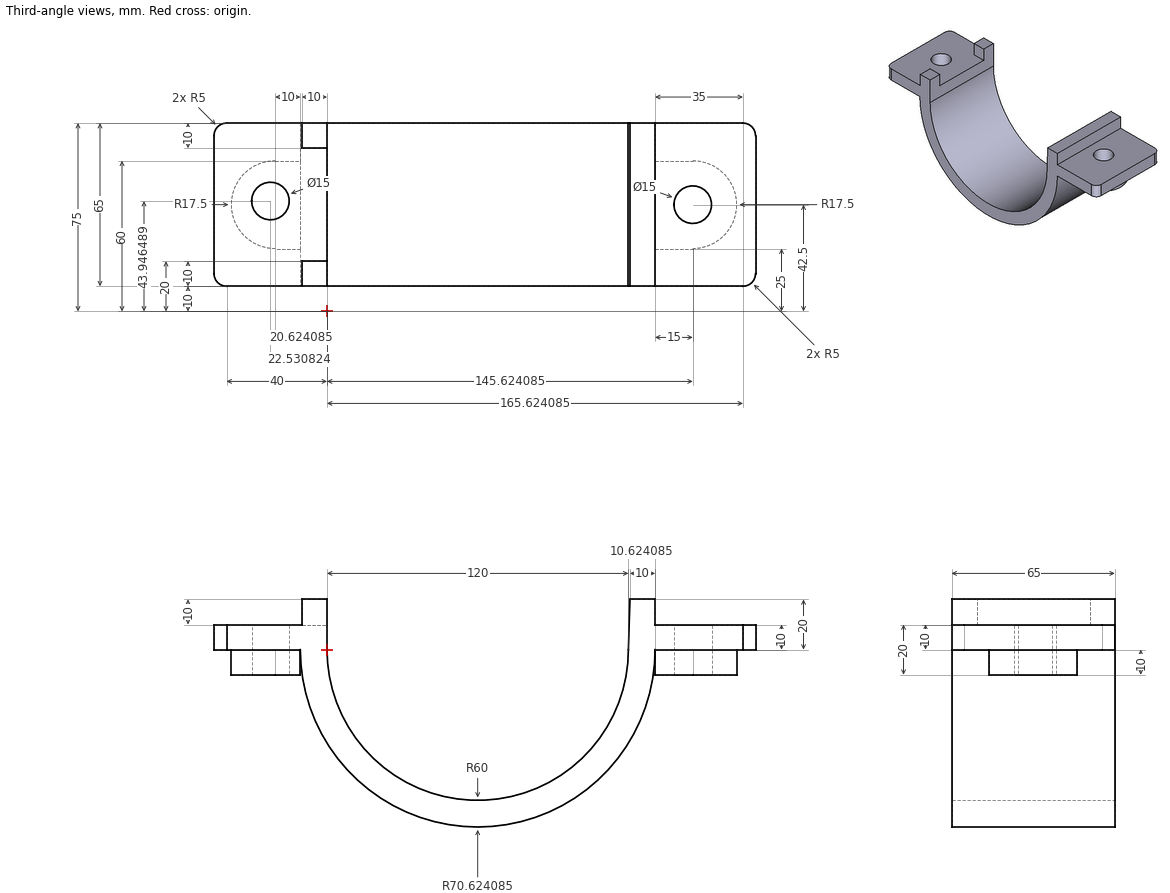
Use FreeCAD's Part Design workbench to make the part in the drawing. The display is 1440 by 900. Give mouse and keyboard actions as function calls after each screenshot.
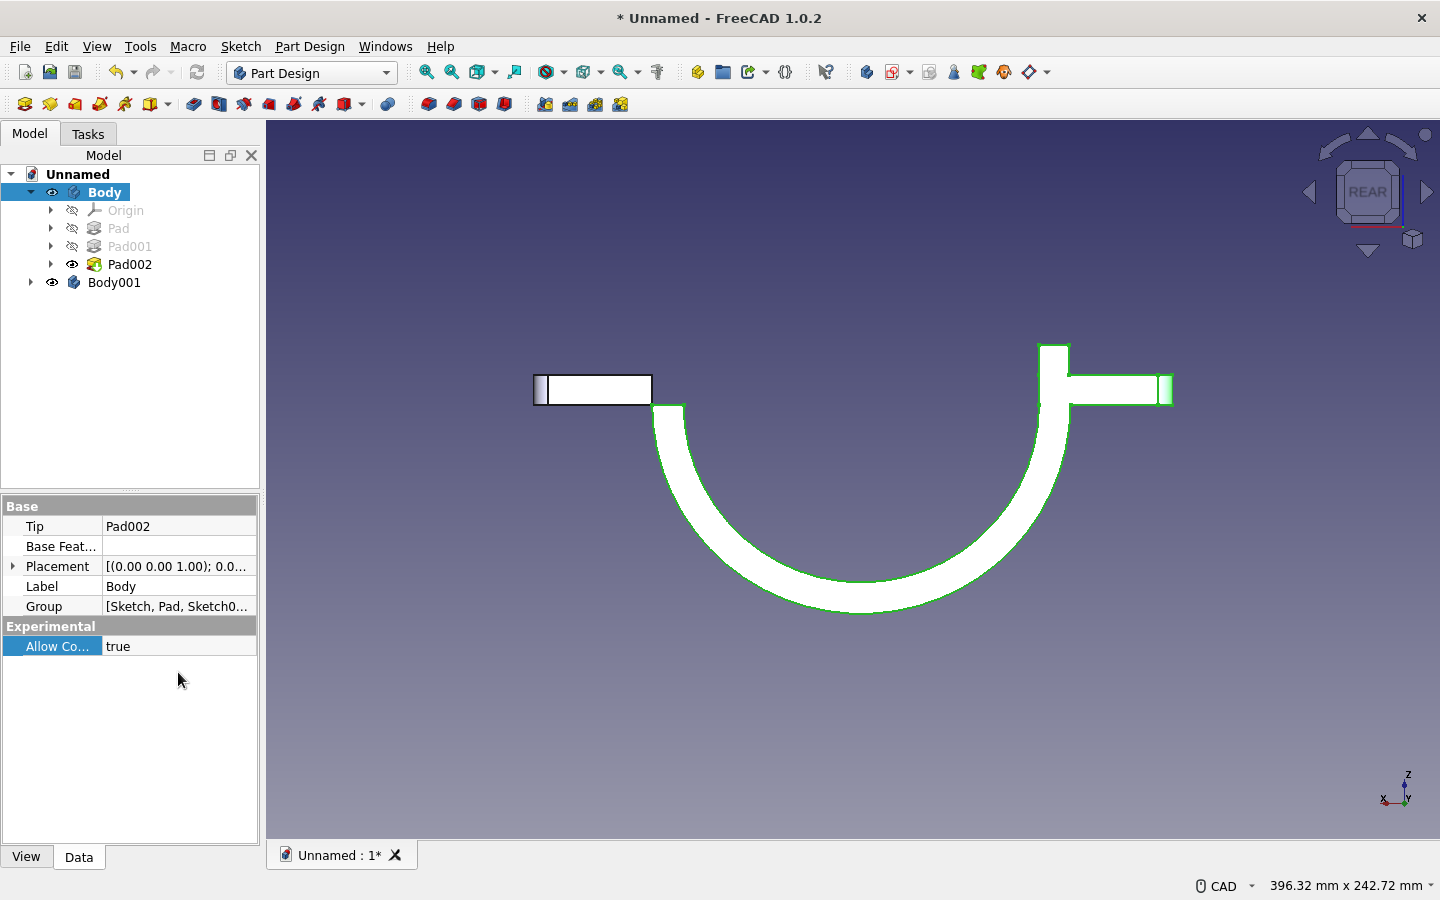
click(97, 282)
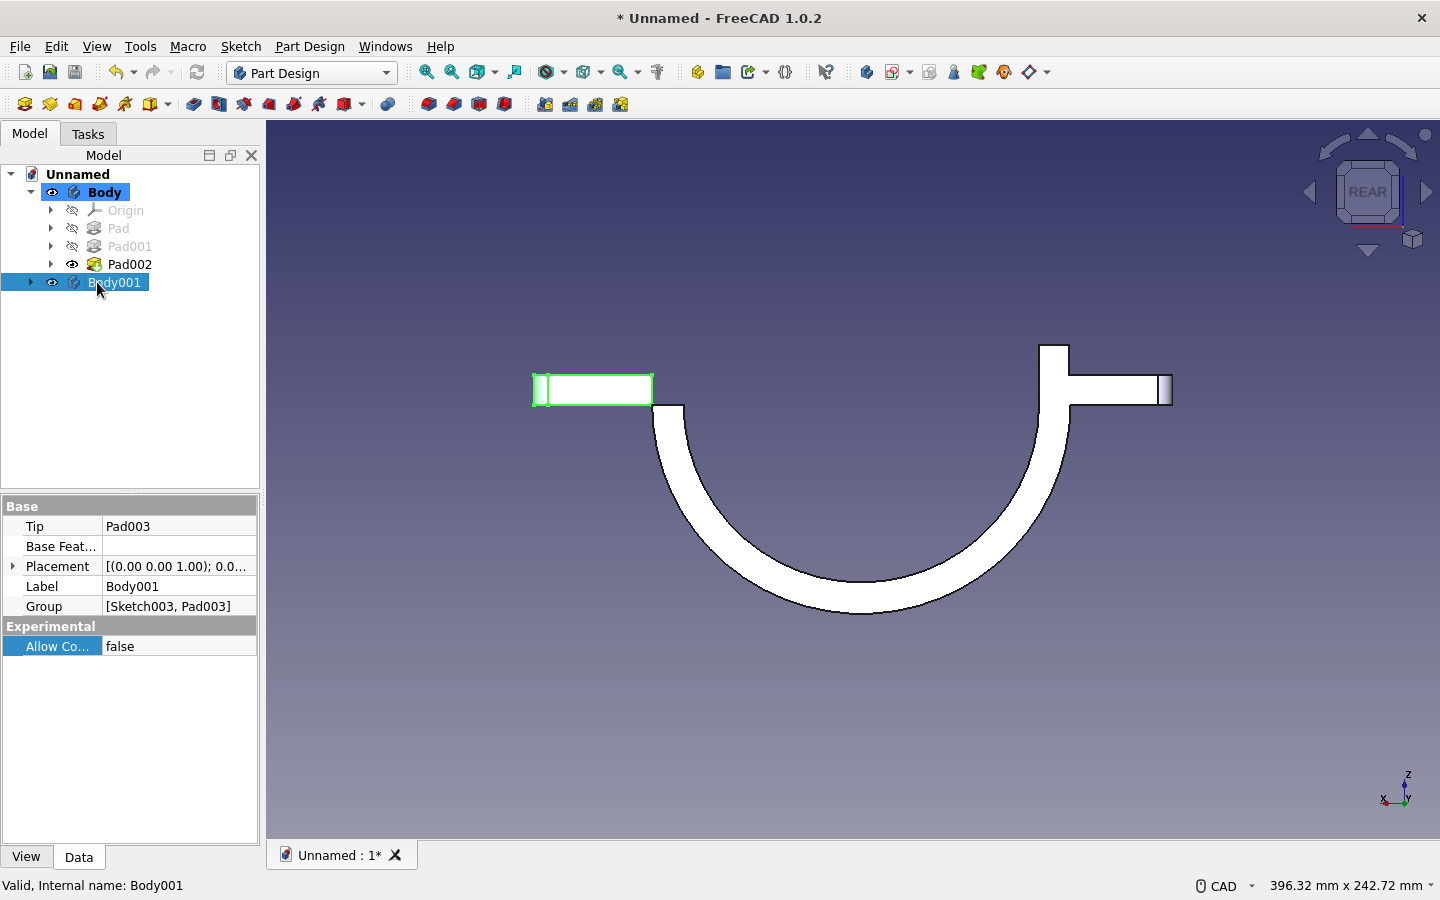
click(388, 104)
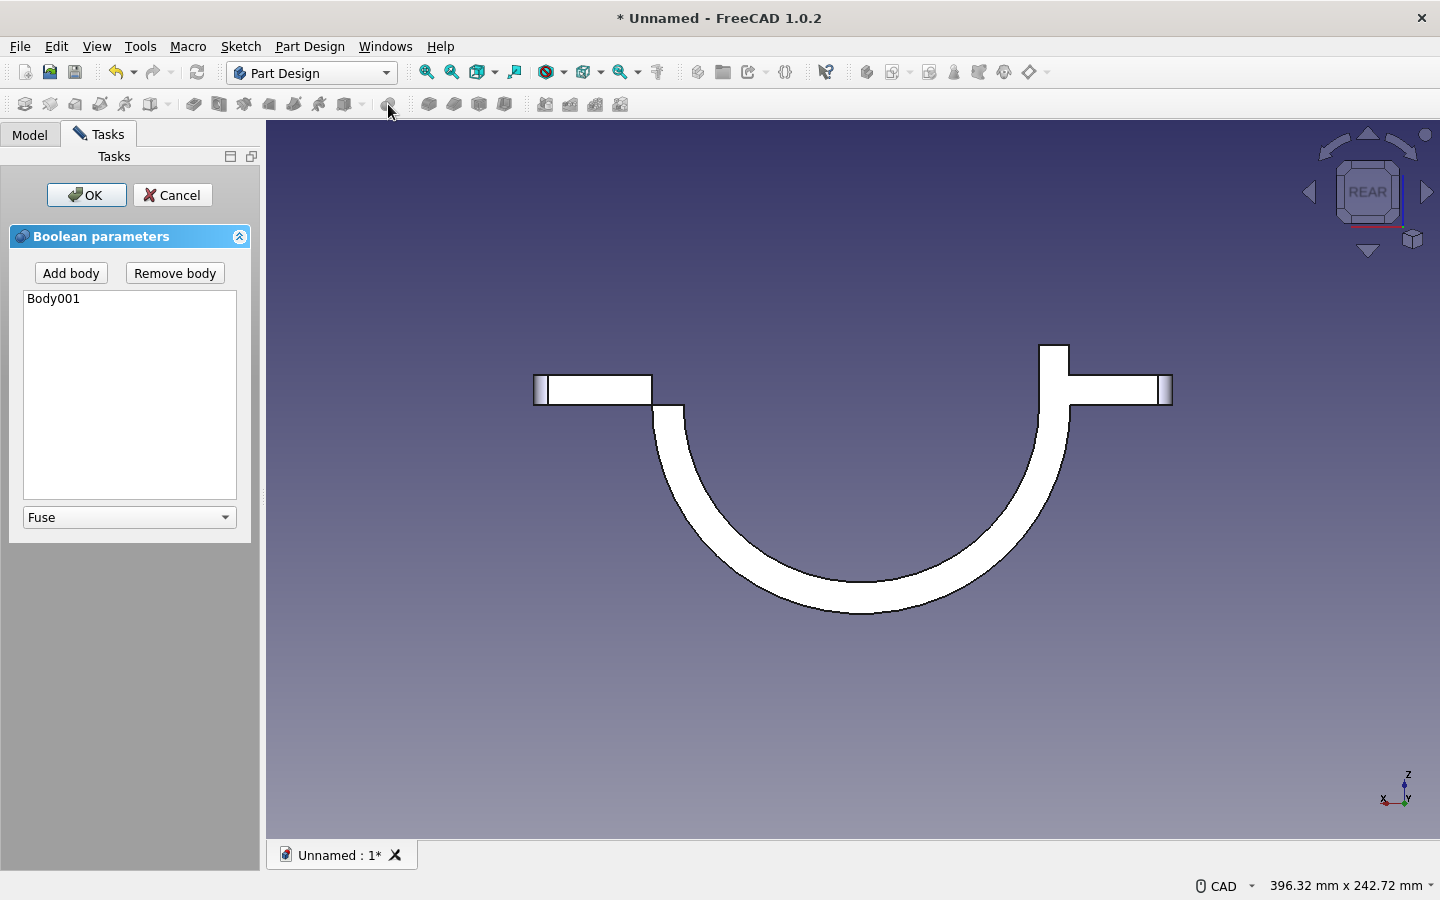
click(87, 195)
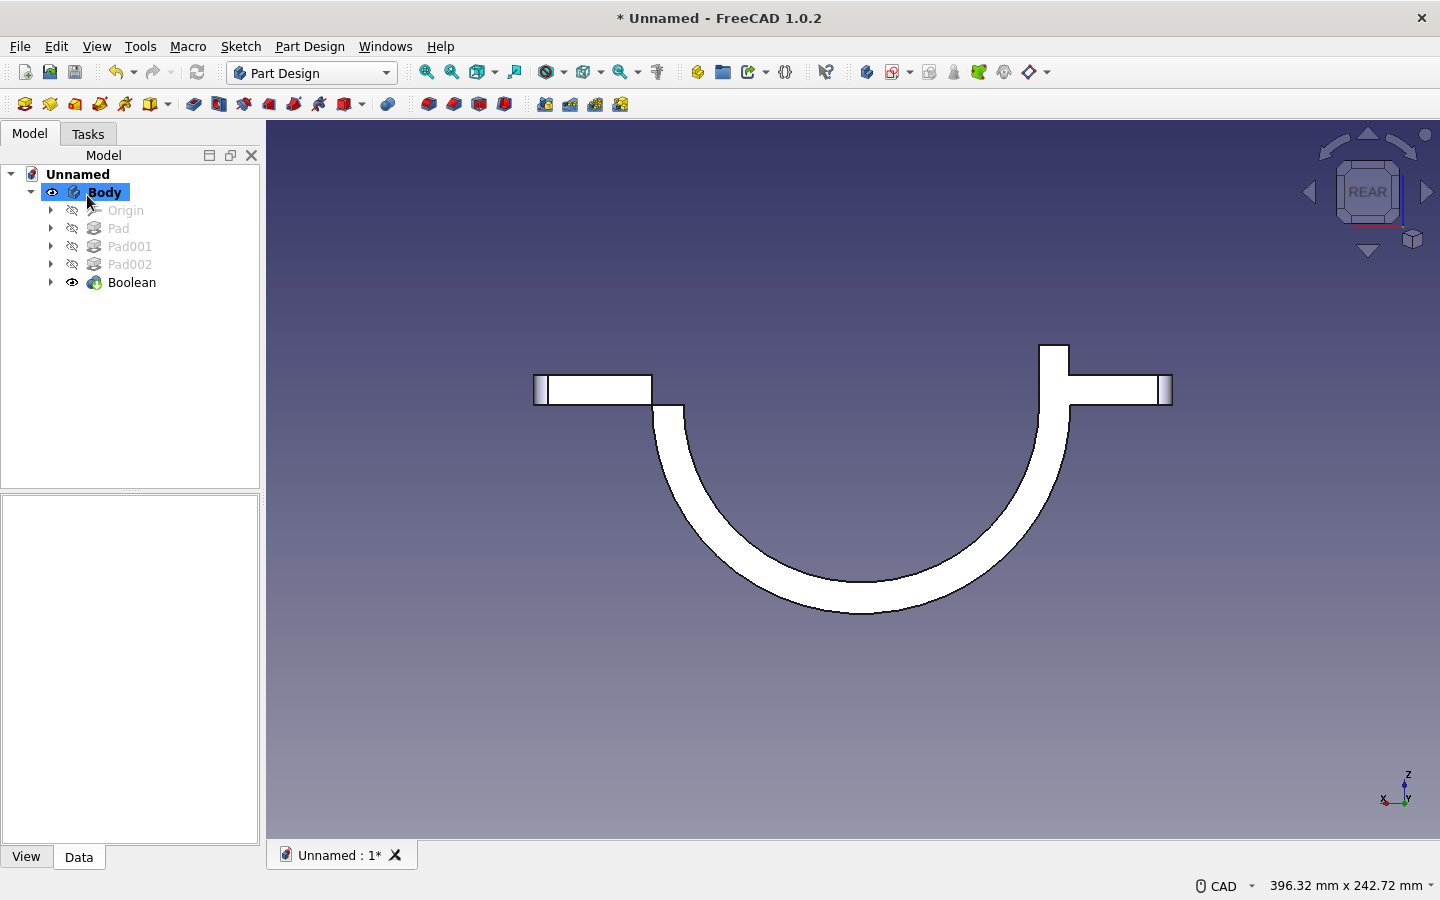
click(833, 594)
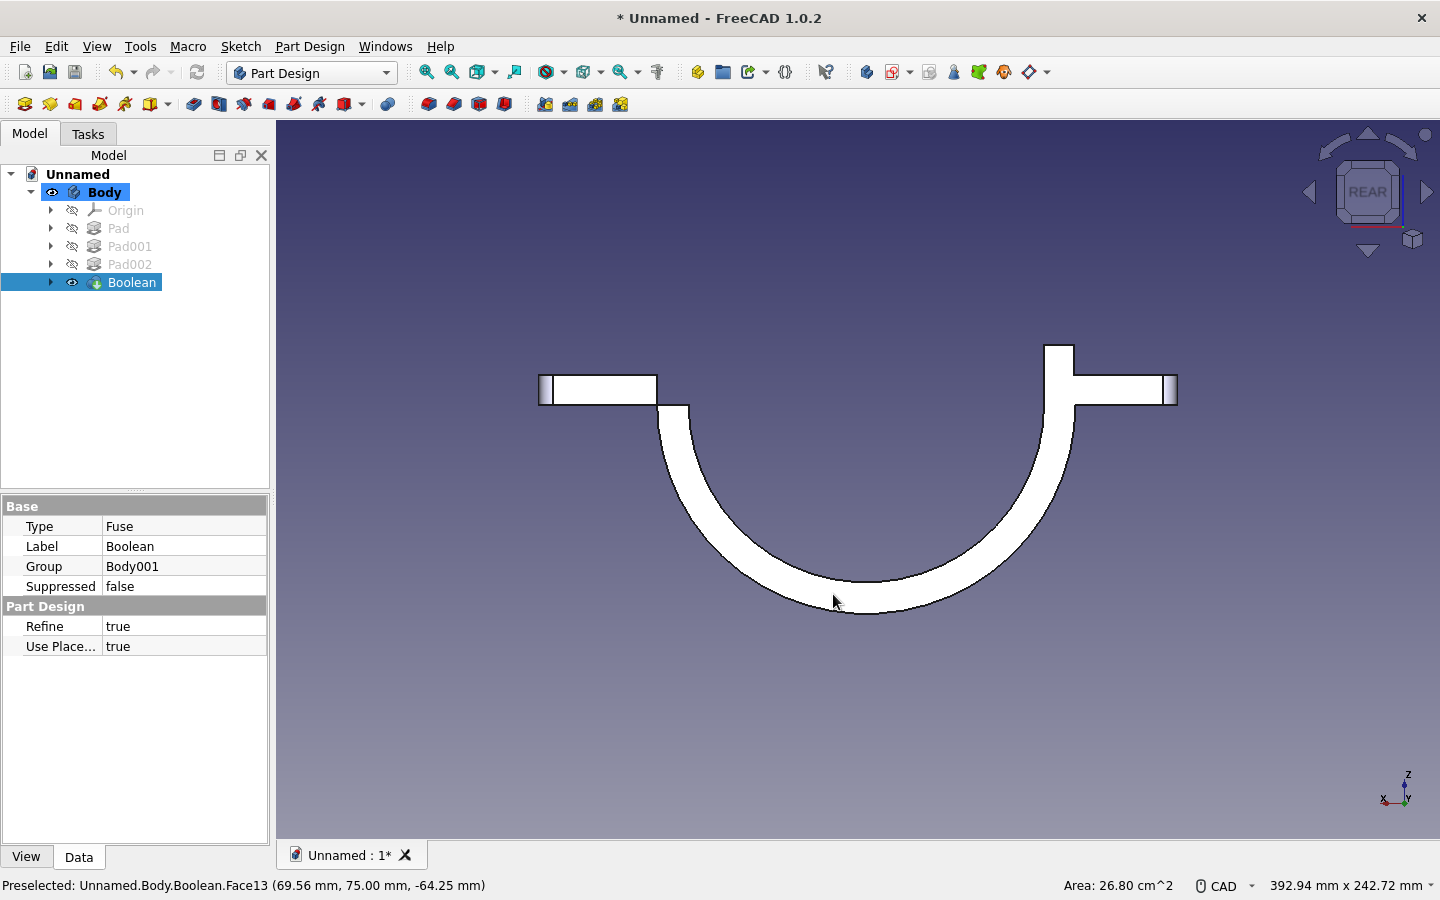
click(892, 72)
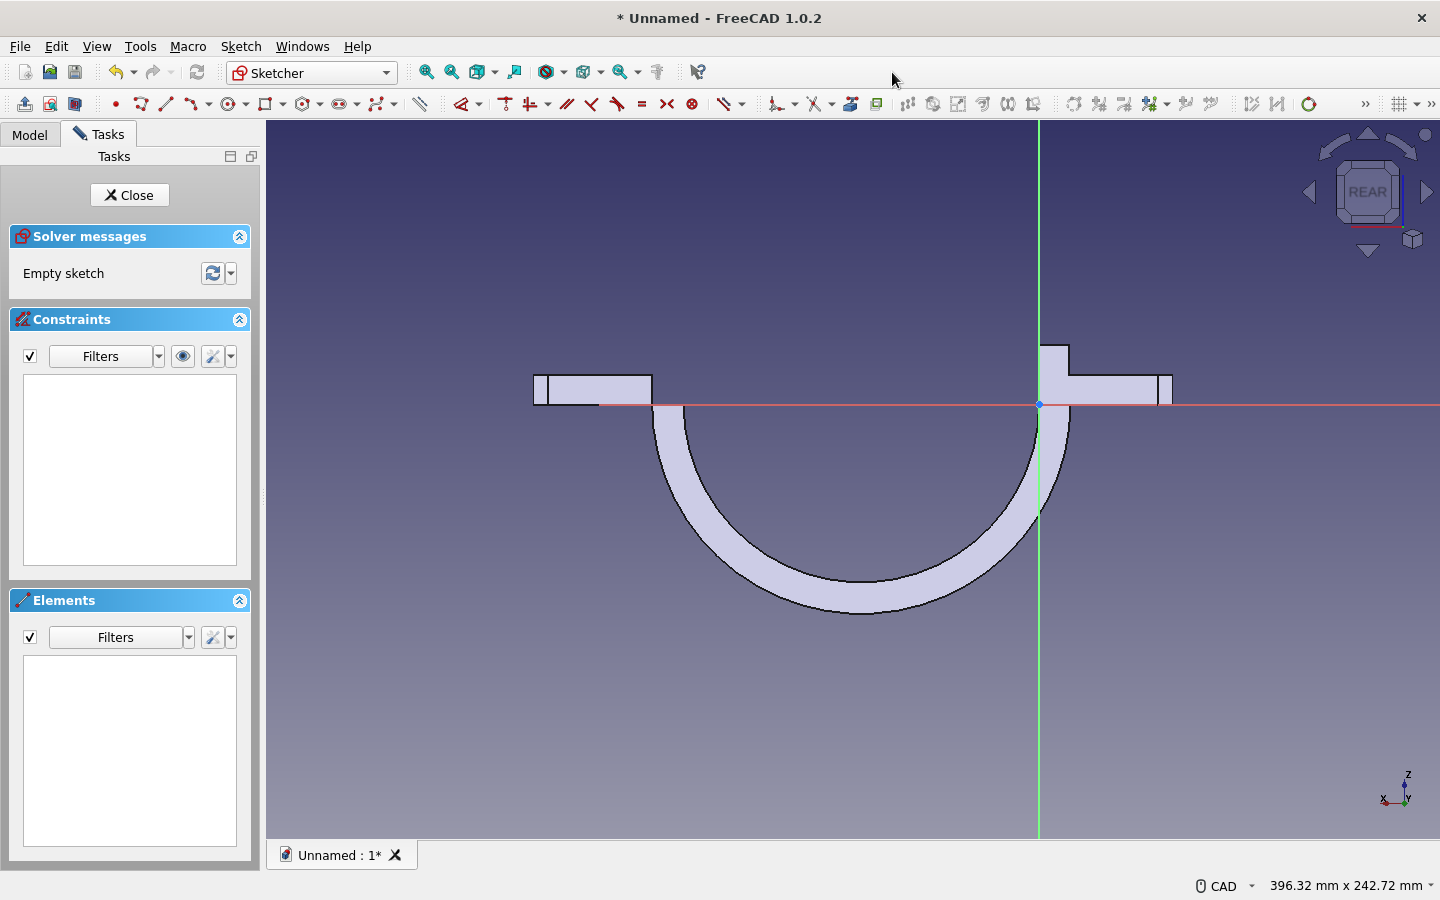
scroll(650, 359, up, 10)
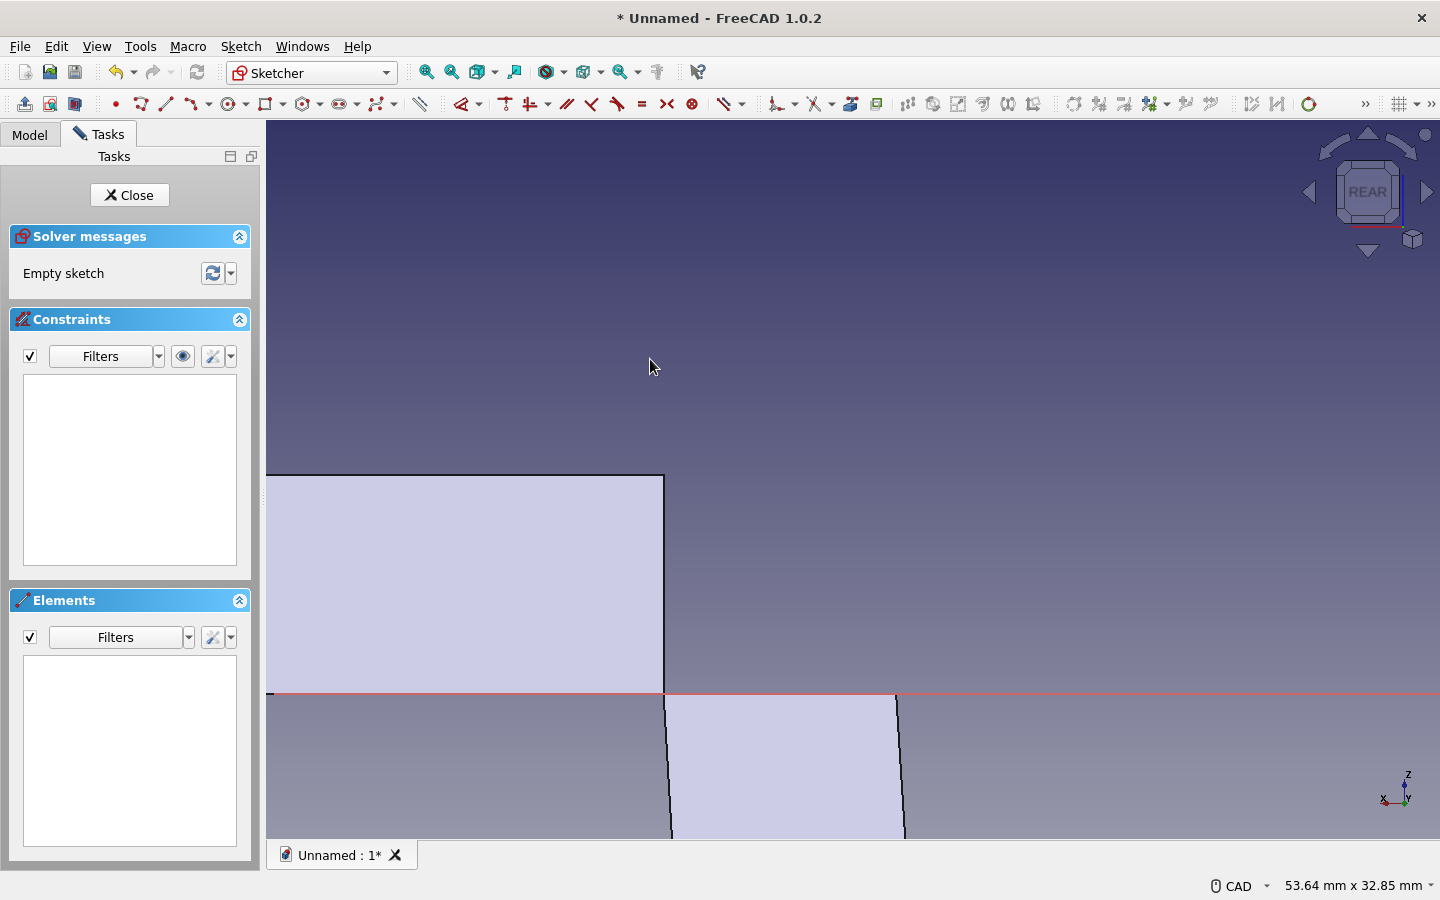
click(141, 104)